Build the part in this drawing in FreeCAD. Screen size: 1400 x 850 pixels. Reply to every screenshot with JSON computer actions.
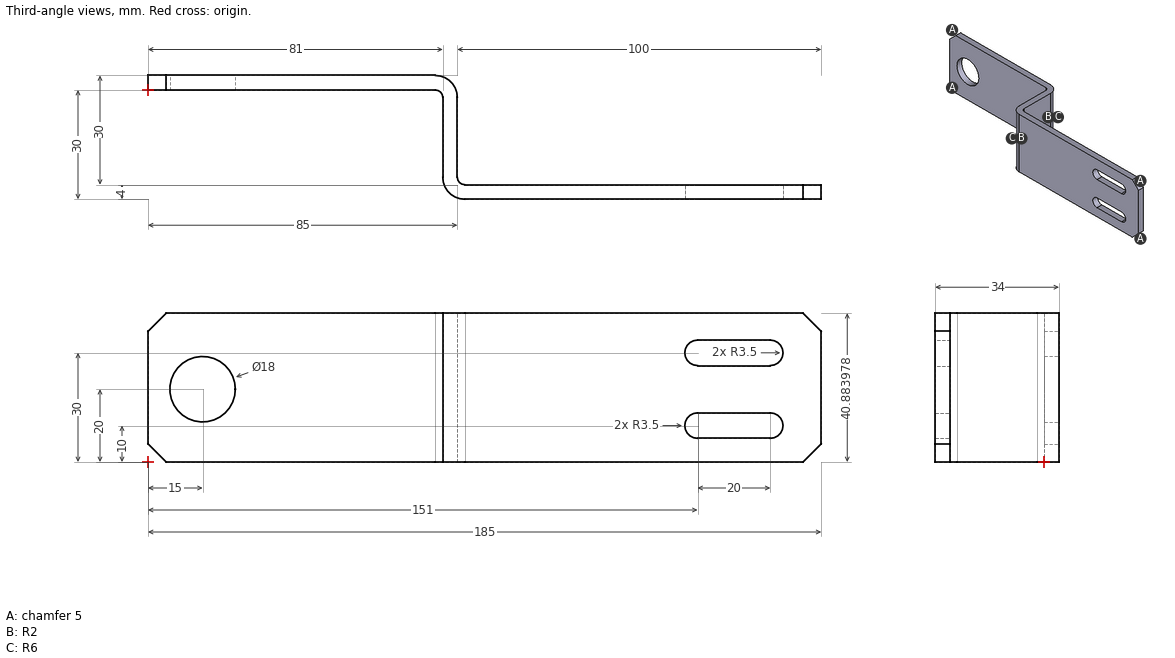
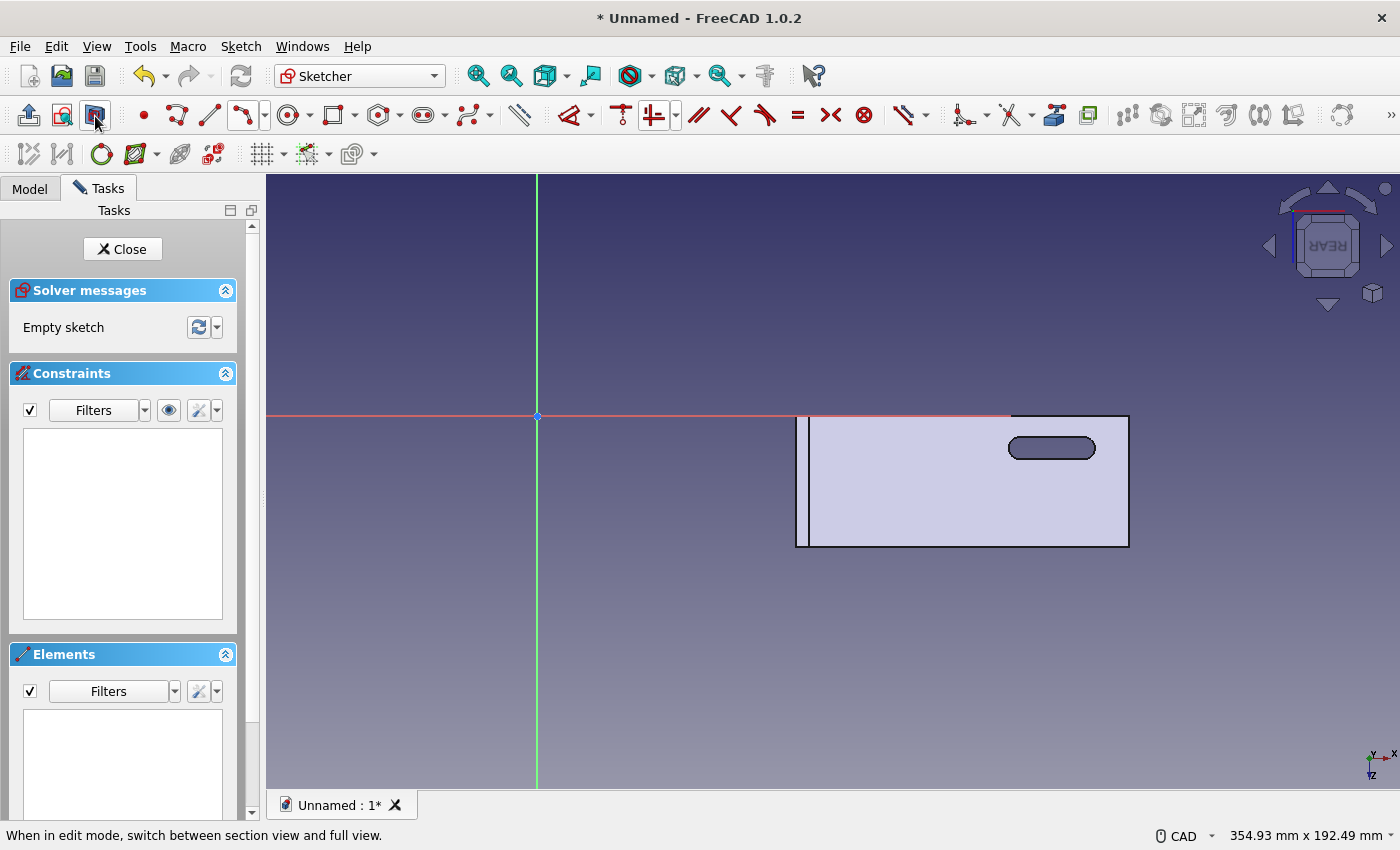
{"action": "scroll", "coordinate": [1097, 517], "scroll_direction": "up", "scroll_amount": 10}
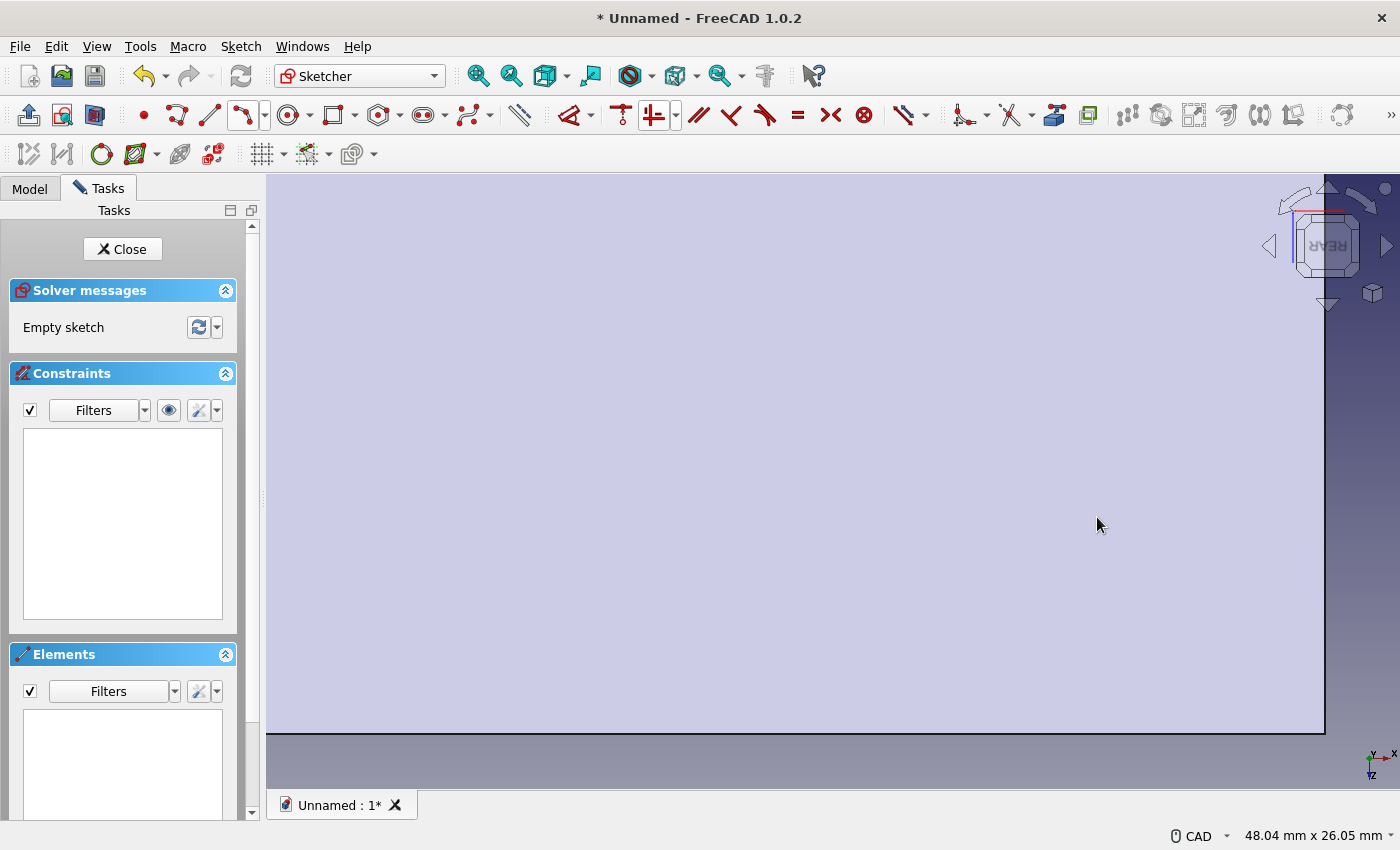
{"action": "left_click", "coordinate": [422, 116]}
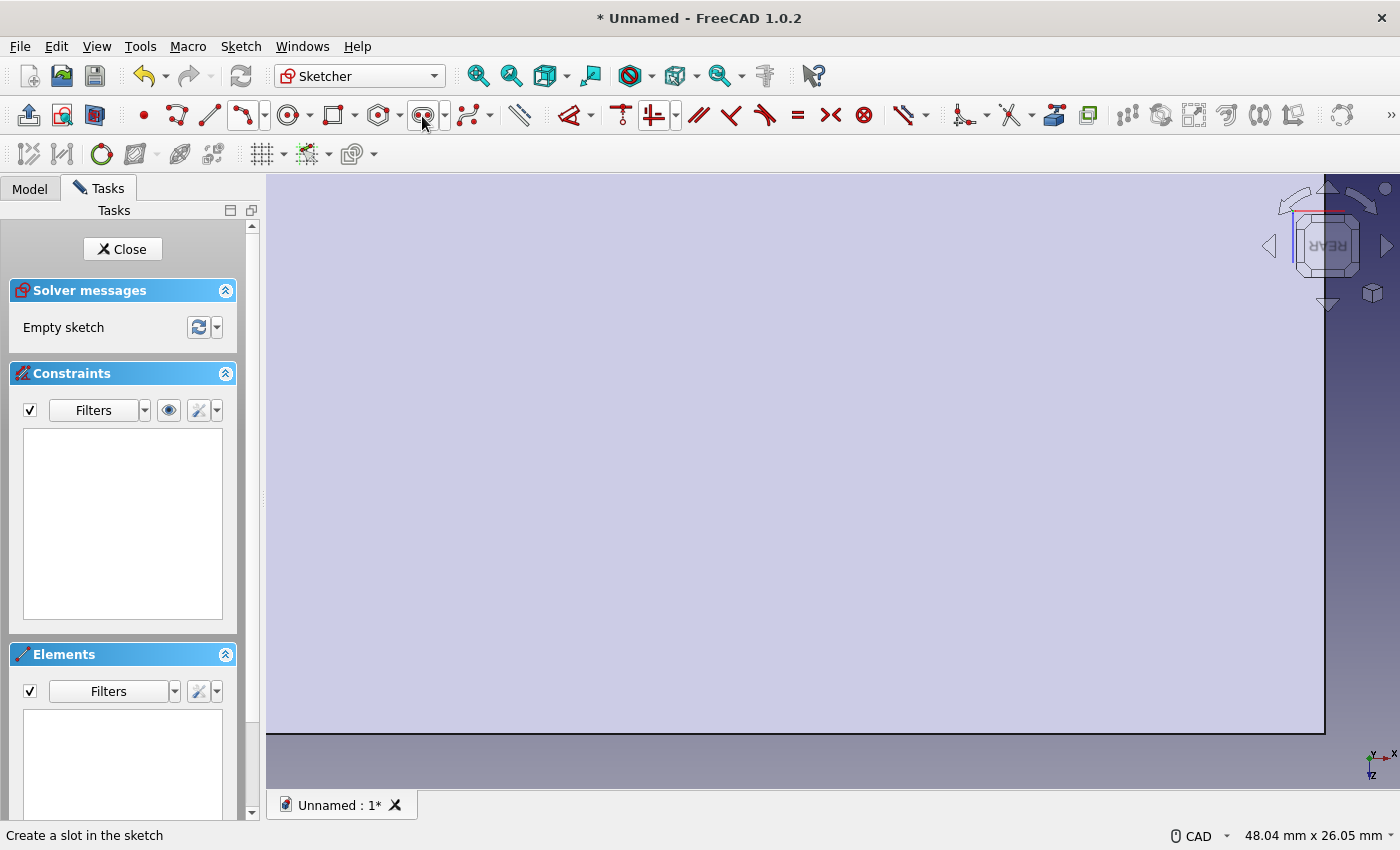
{"action": "left_click", "coordinate": [523, 477]}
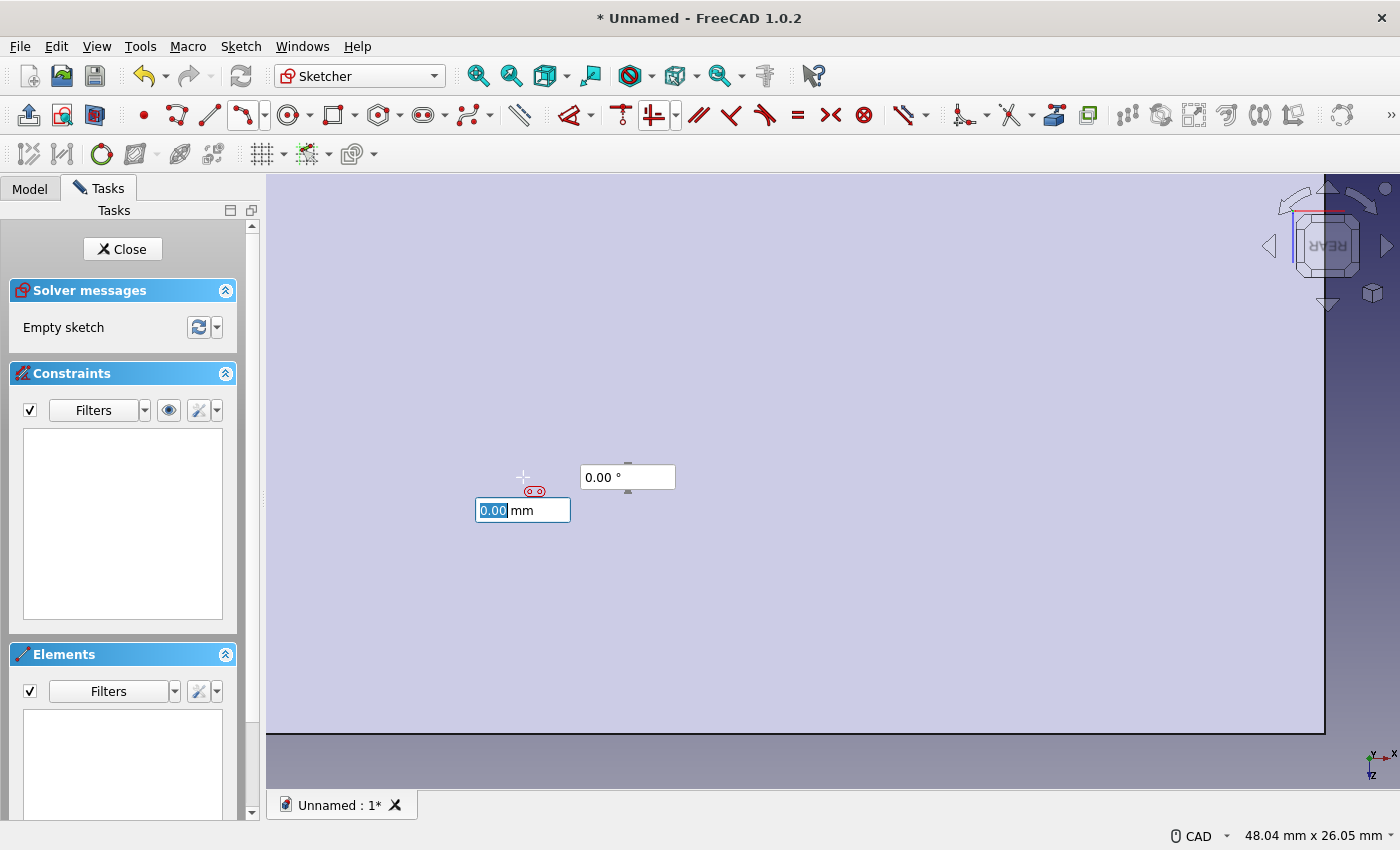
{"action": "left_click", "coordinate": [995, 477]}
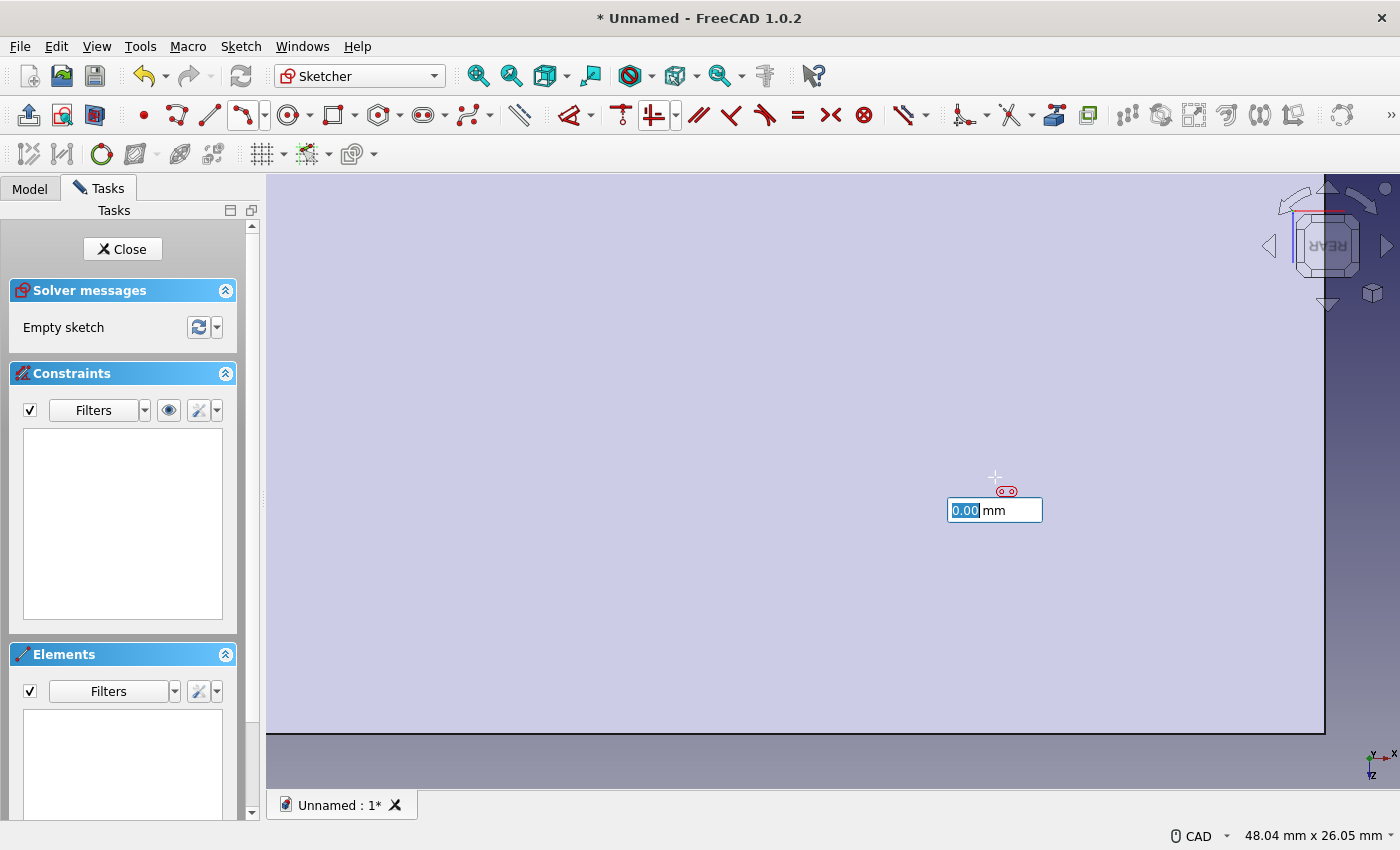
{"action": "left_click", "coordinate": [759, 559]}
{"action": "key", "text": "Escape"}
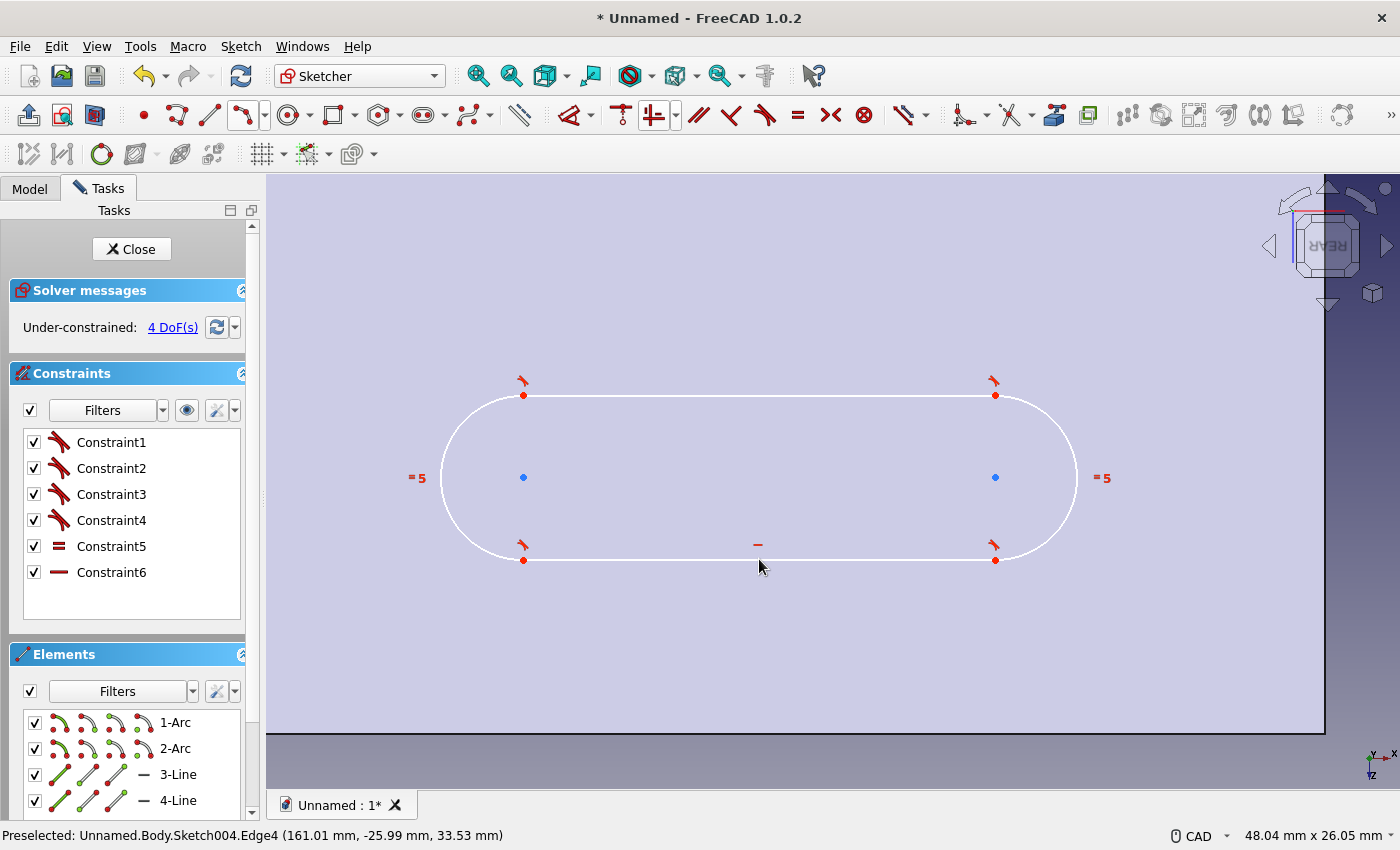
{"action": "left_click", "coordinate": [568, 116]}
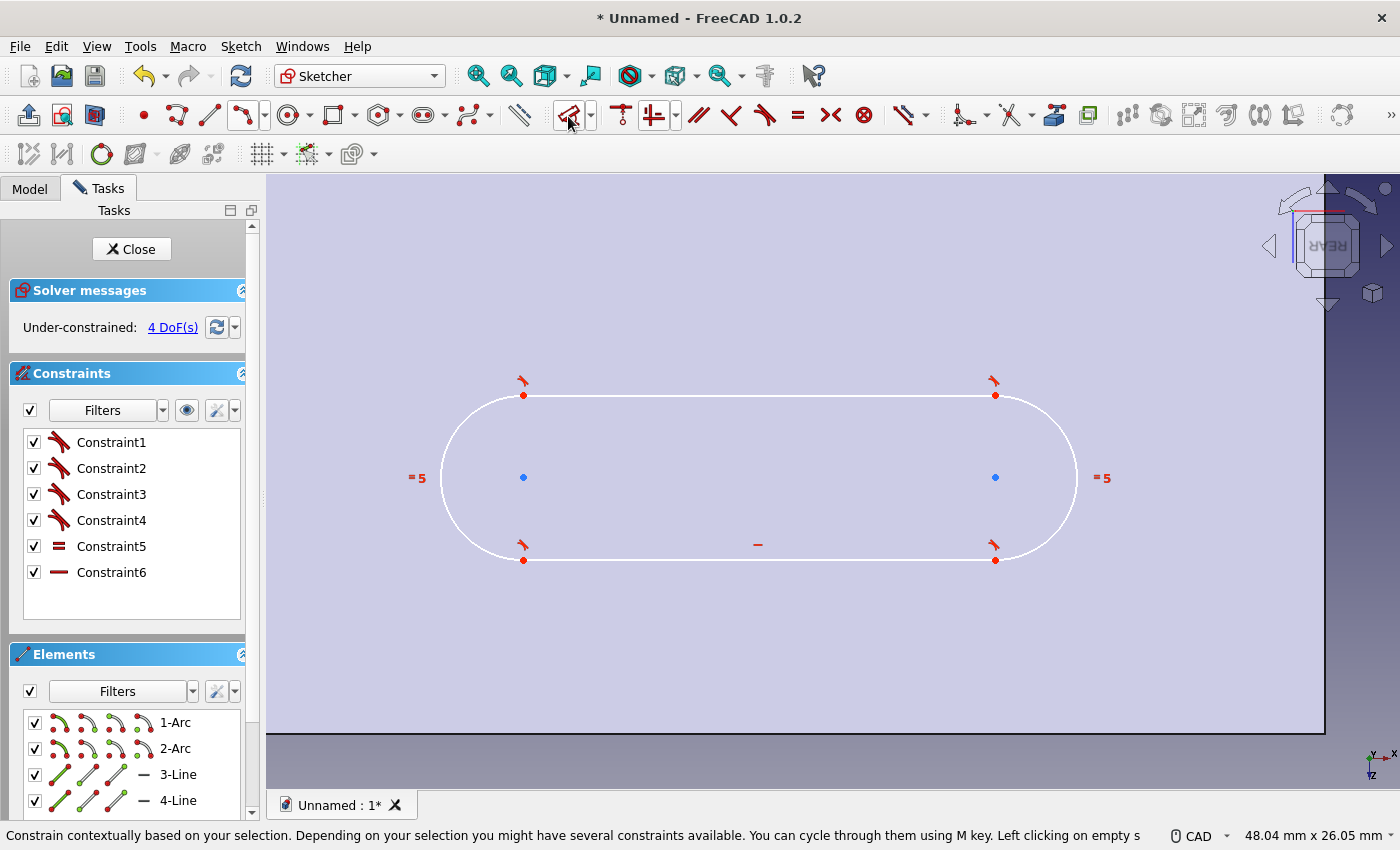
{"action": "left_click", "coordinate": [457, 430]}
{"action": "left_click", "coordinate": [431, 411]}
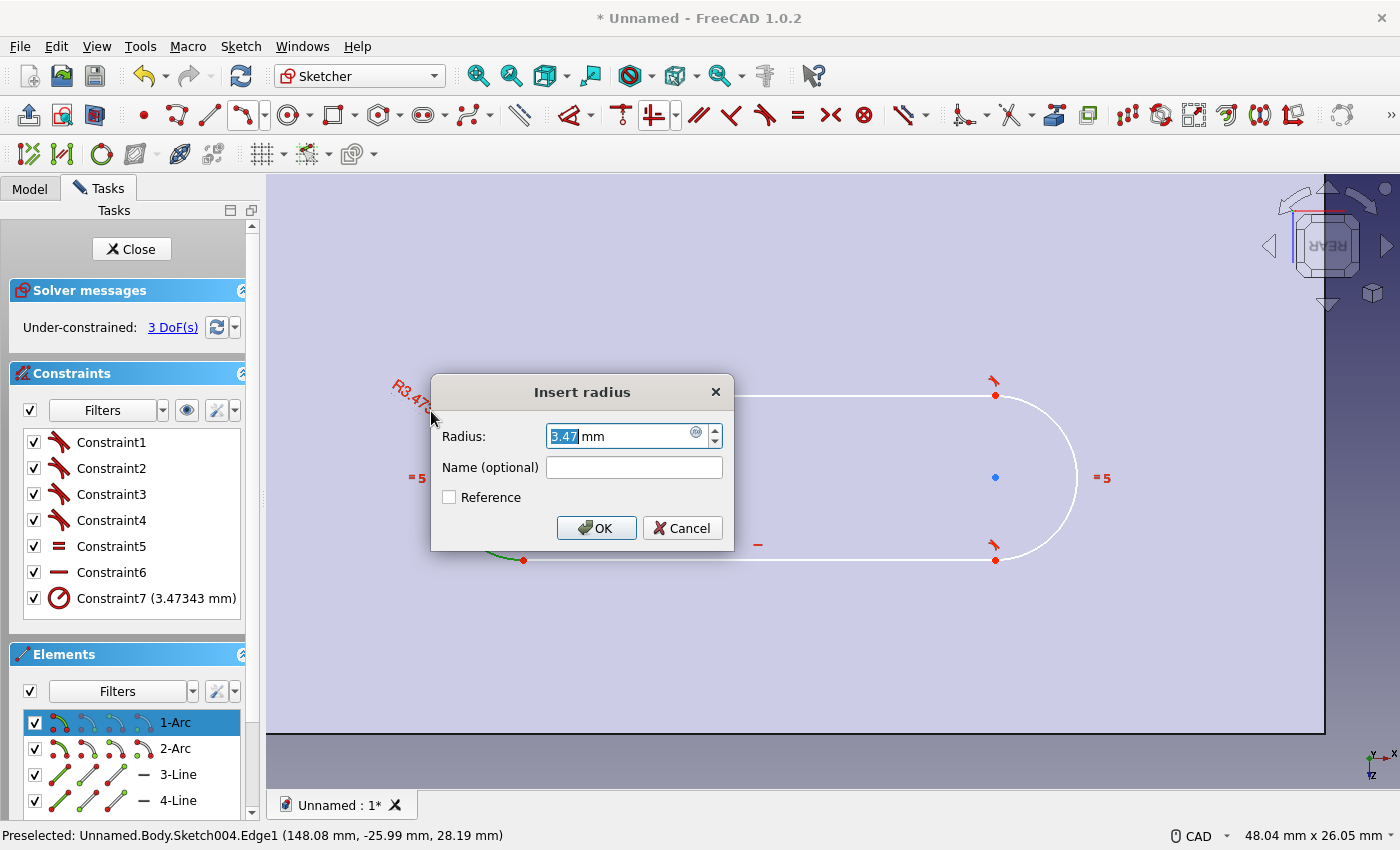
{"action": "type", "text": "3.5"}
{"action": "key", "text": "Return"}